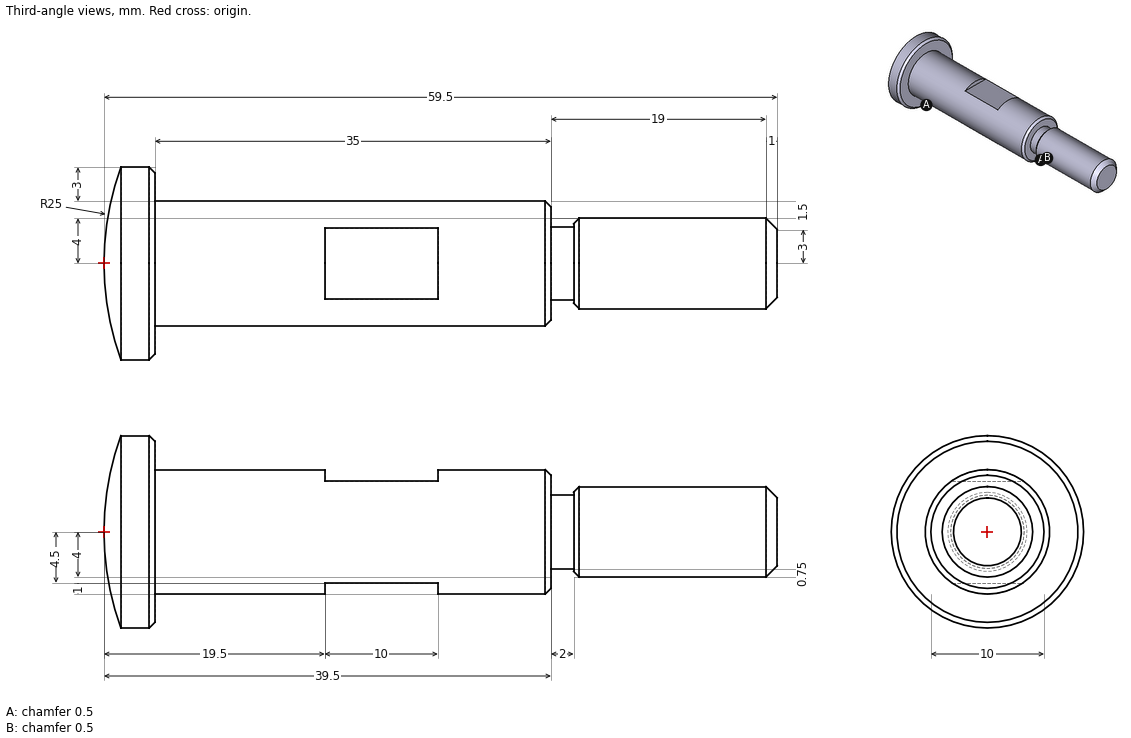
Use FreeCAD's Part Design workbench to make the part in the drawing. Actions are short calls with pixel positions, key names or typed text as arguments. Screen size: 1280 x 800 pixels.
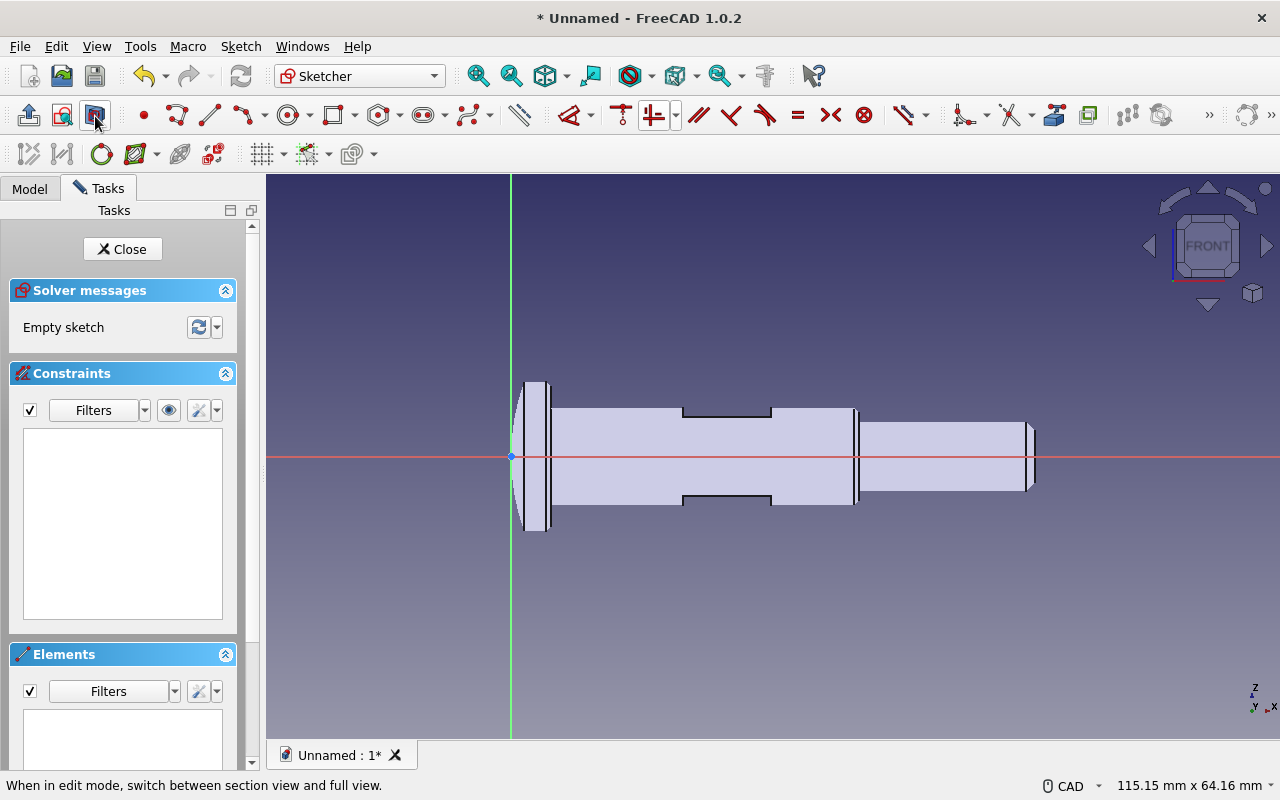
scroll(876, 490, up, 15)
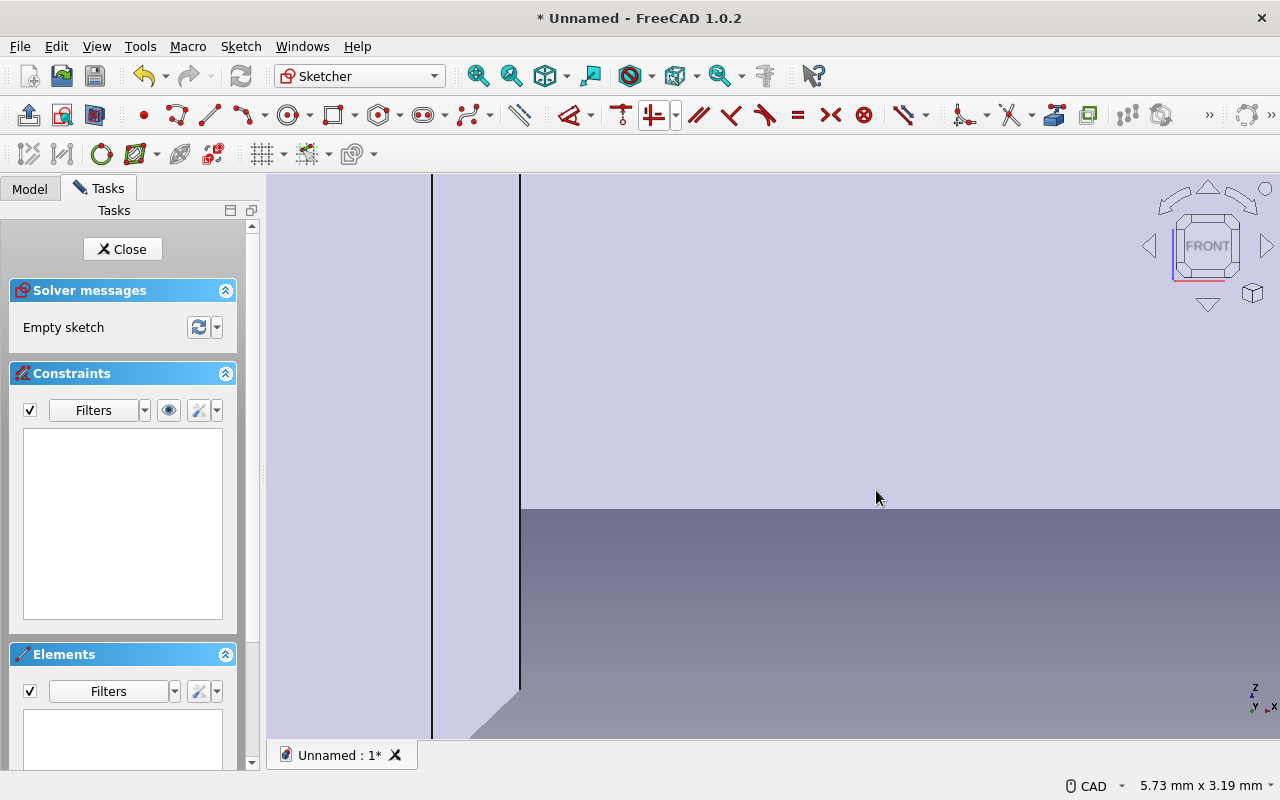
scroll(682, 430, up, 2)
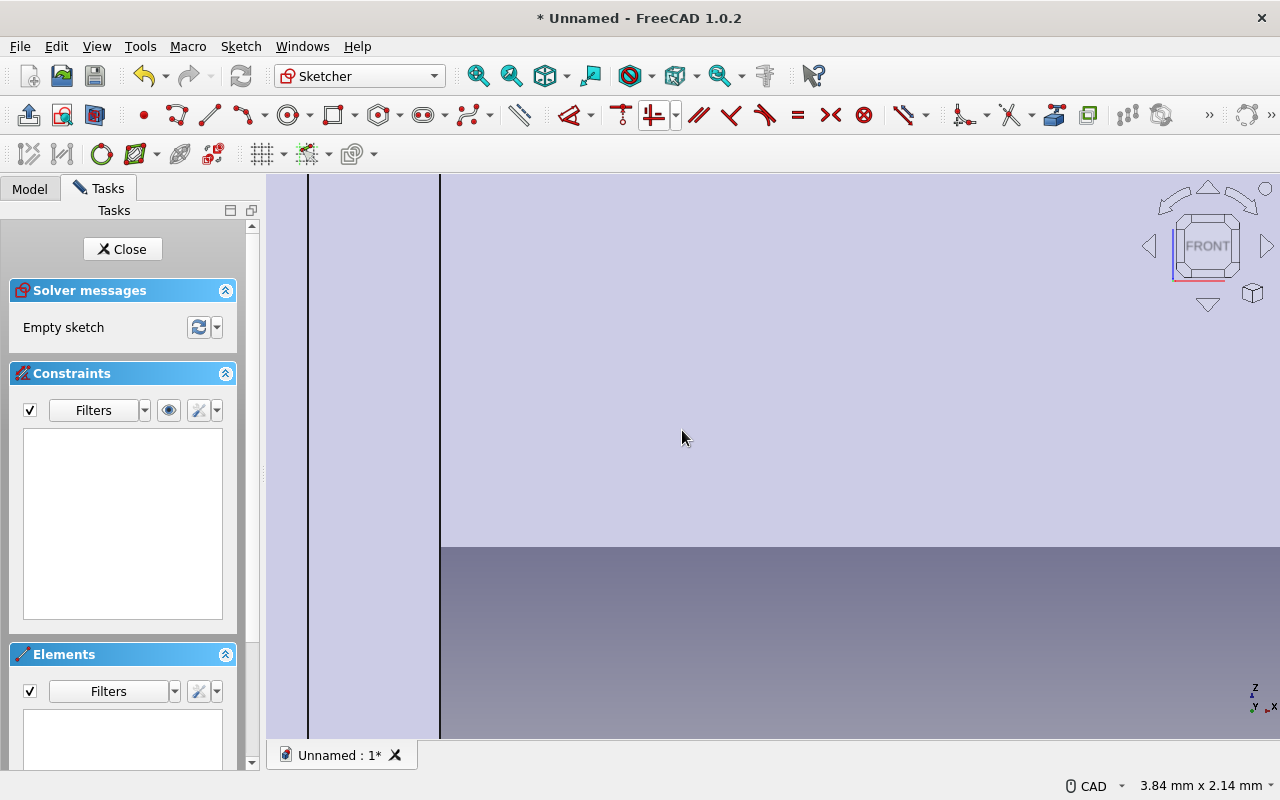
click(332, 116)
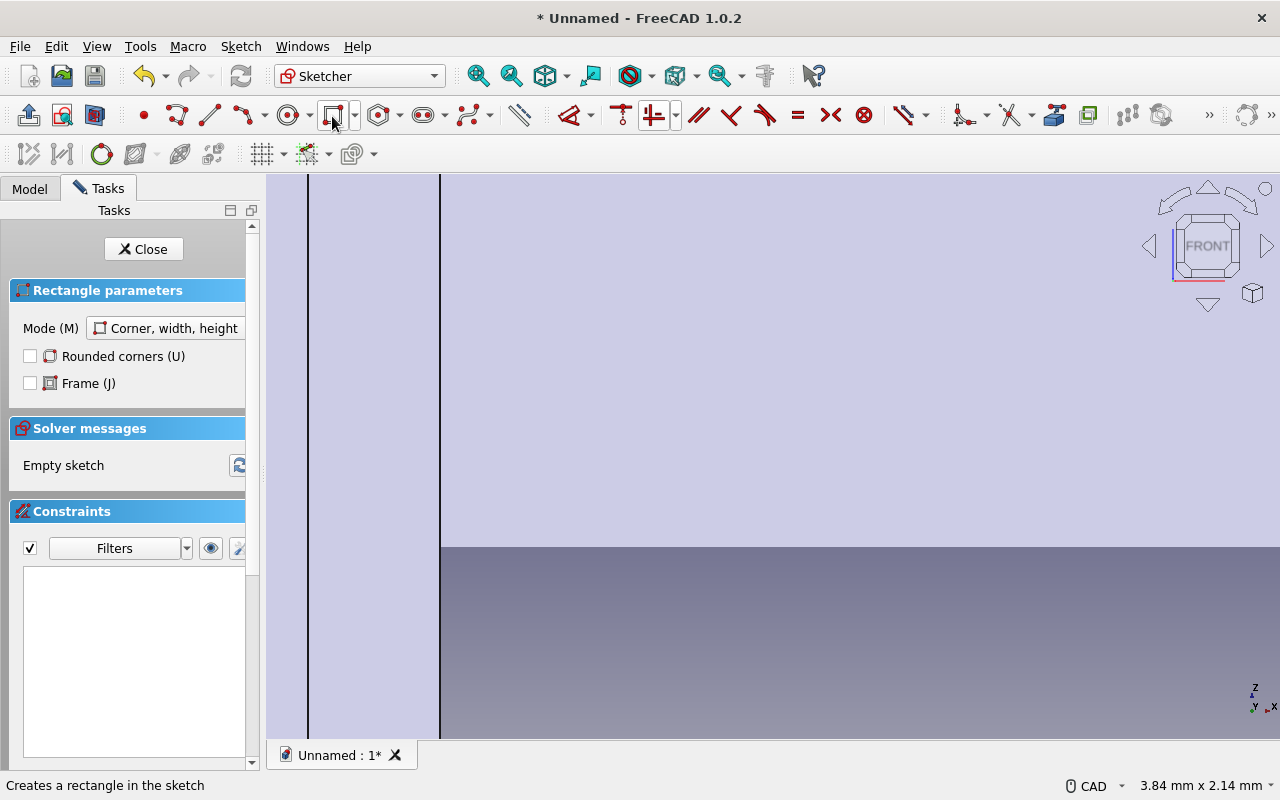
click(440, 357)
move(968, 555)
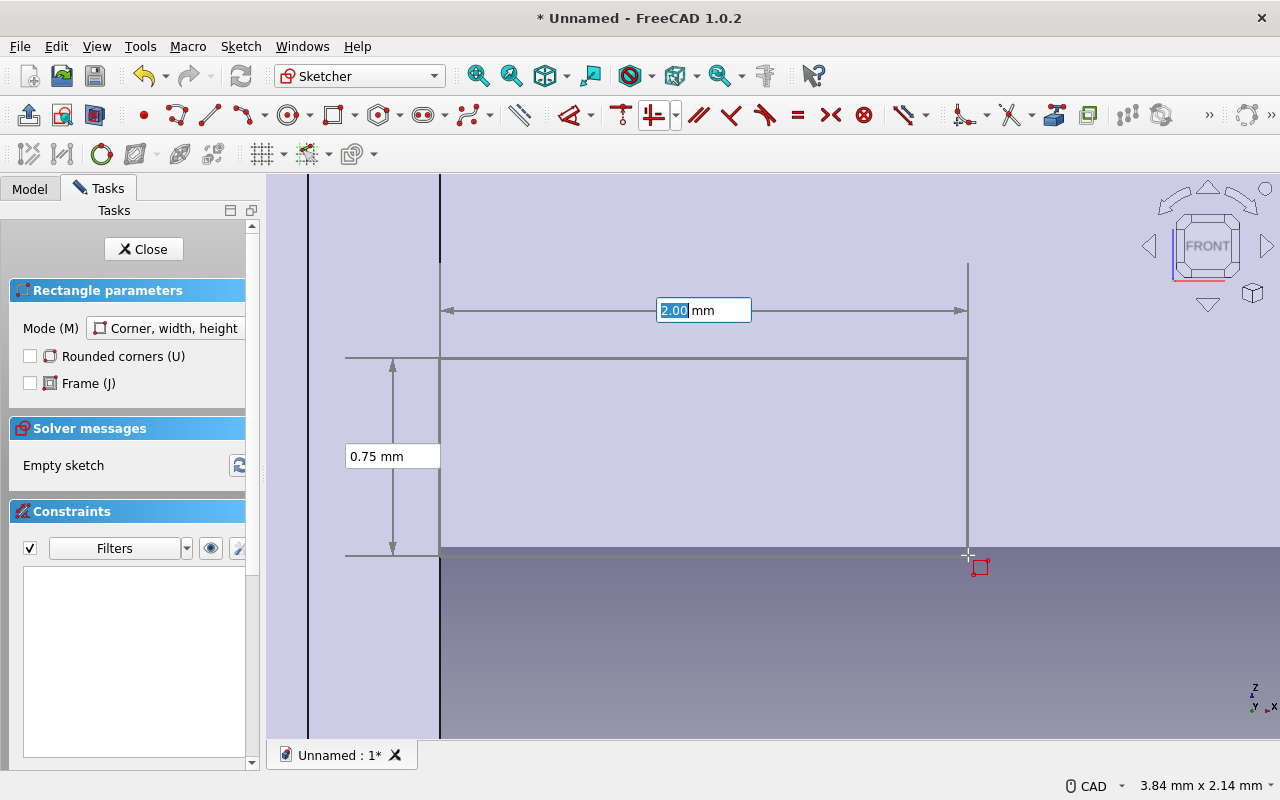
text(2)
key(Tab)
text(0.75)
key(Return)
key(Escape)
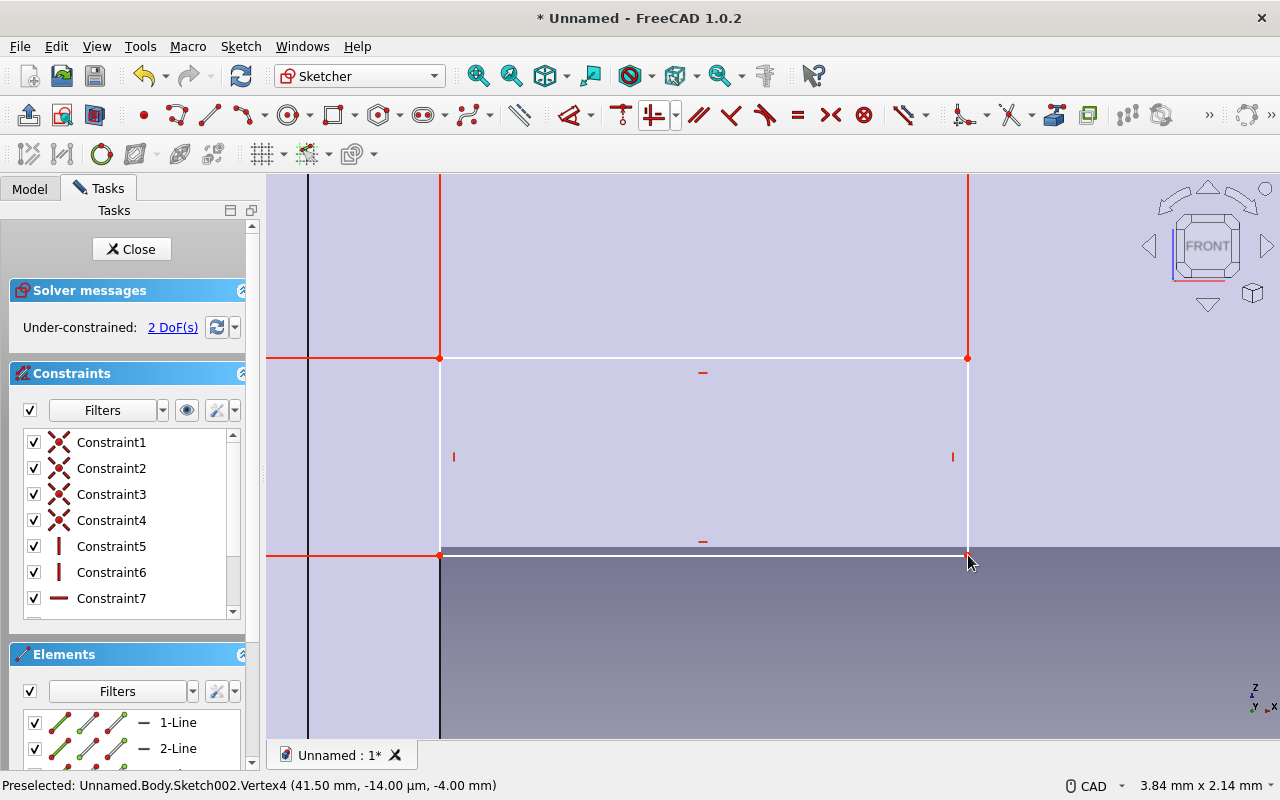
click(568, 116)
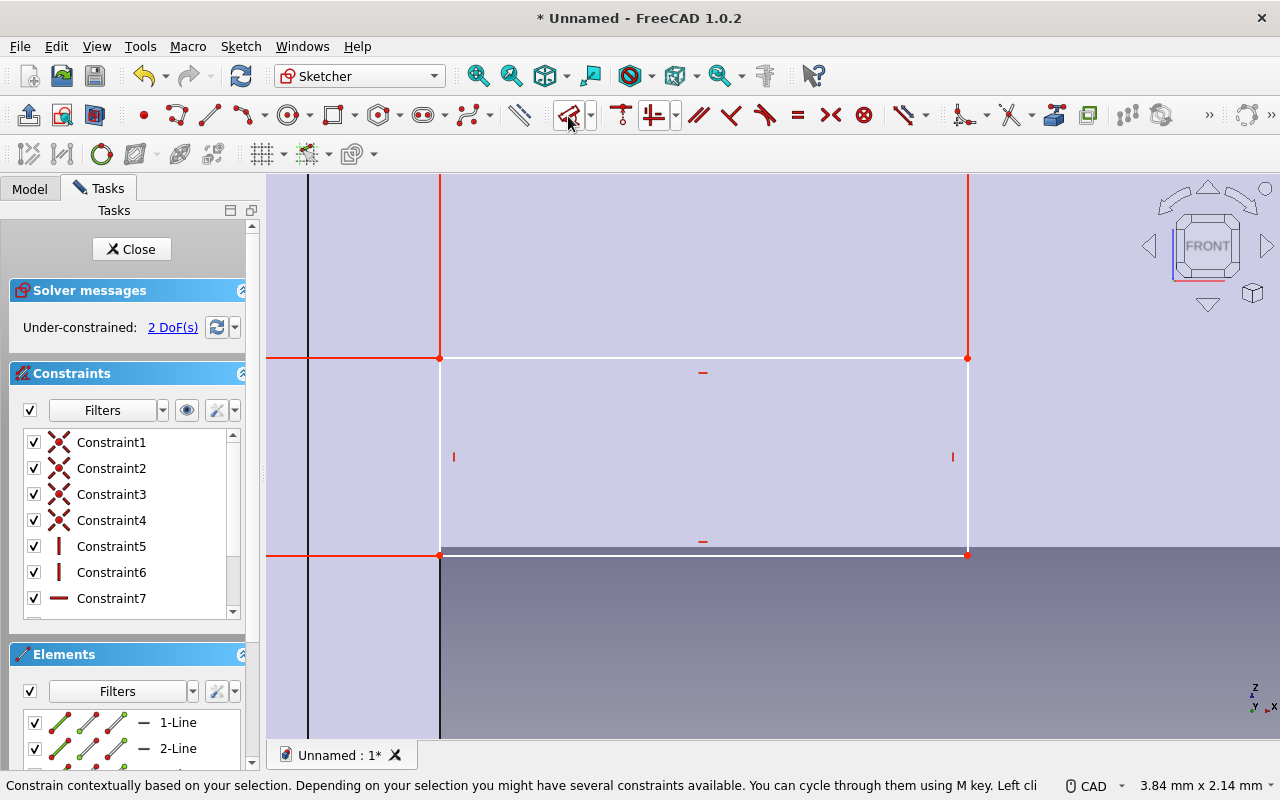
click(440, 556)
click(474, 379)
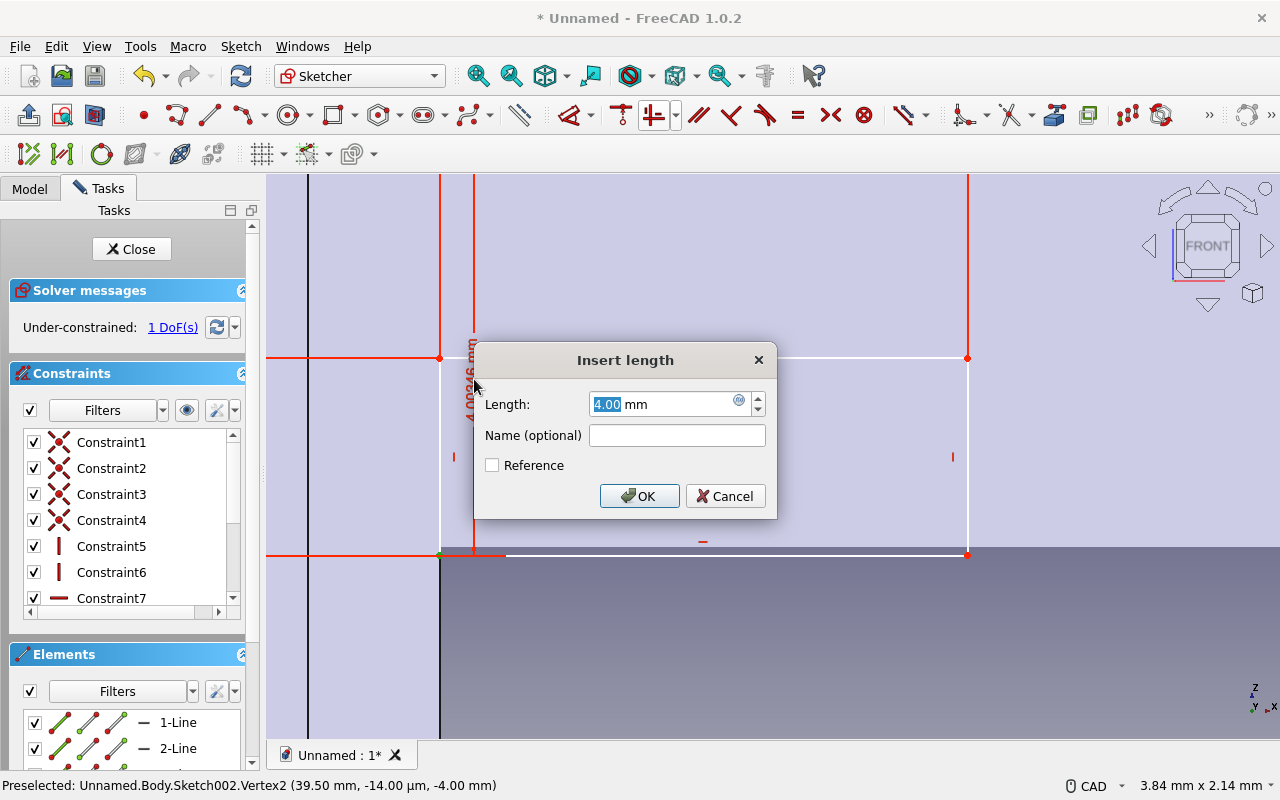
text(4)
key(Return)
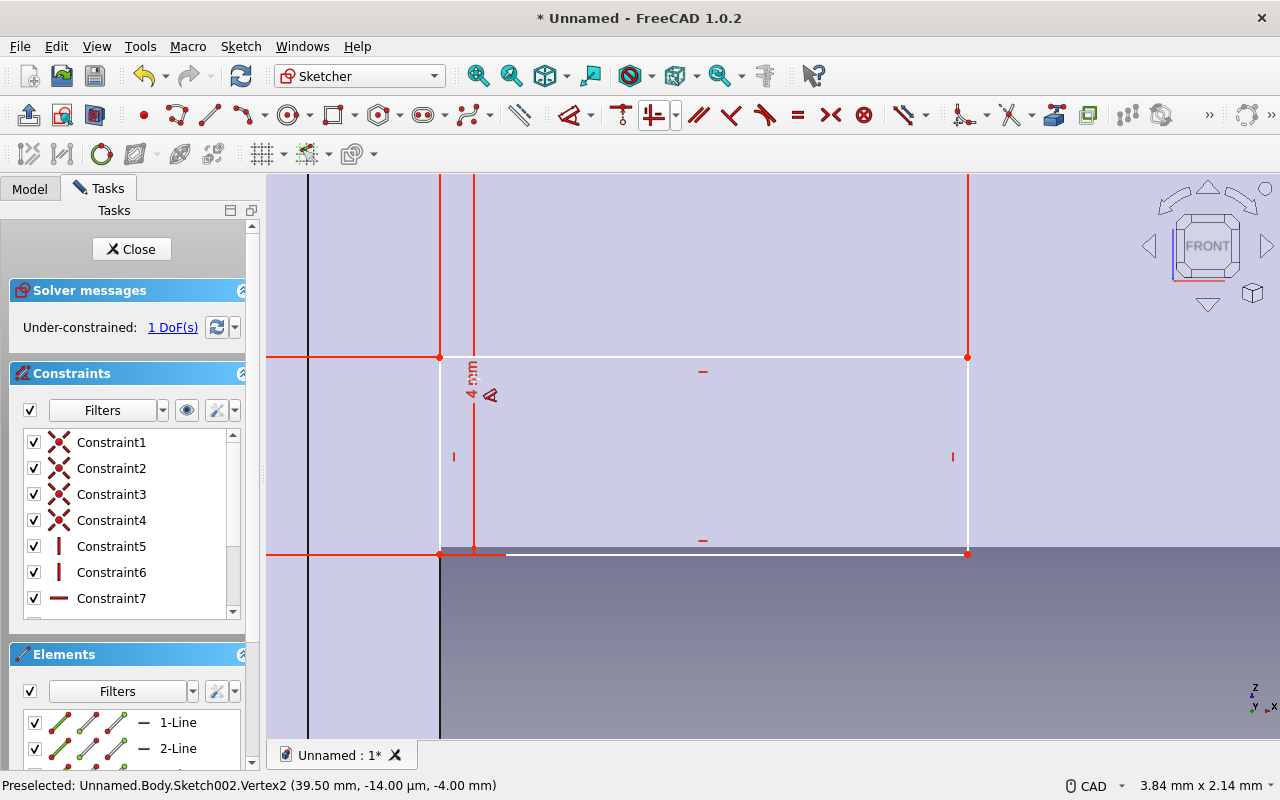
click(440, 357)
click(367, 391)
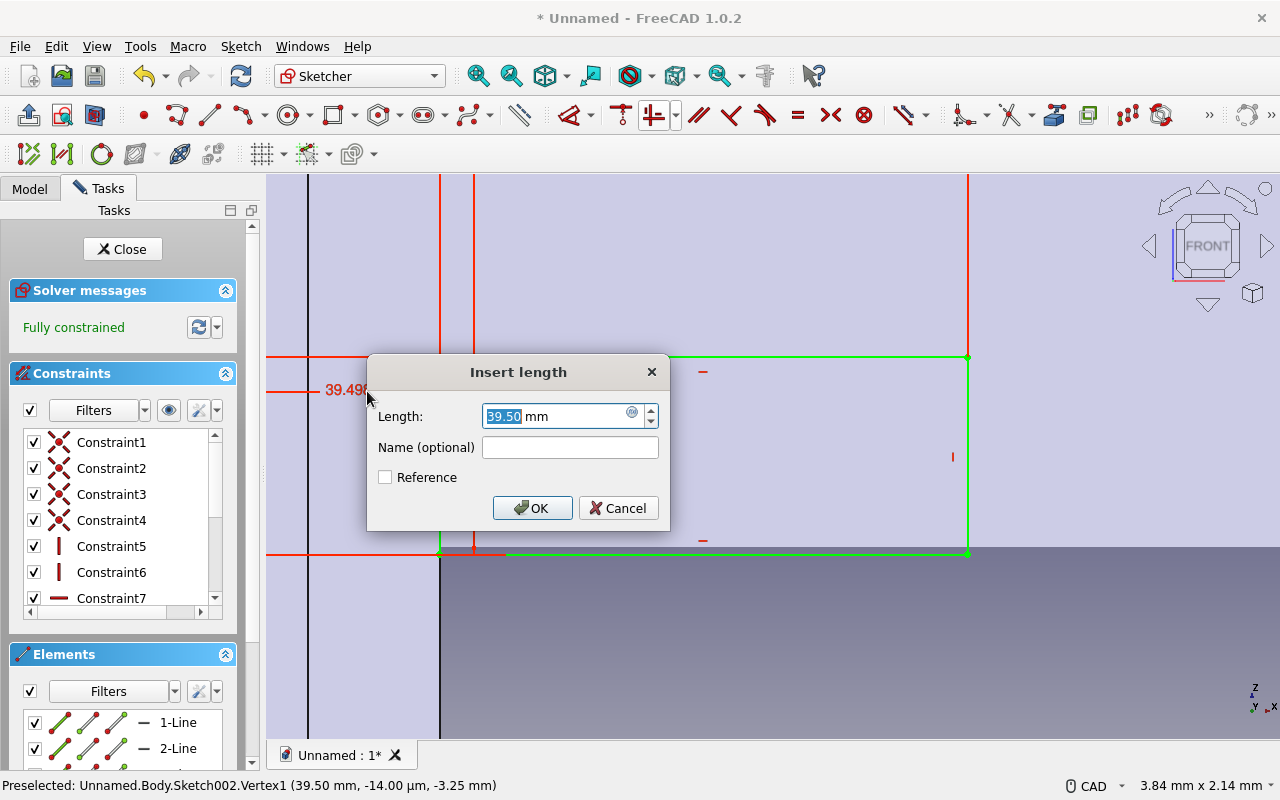
text(39.5)
key(Return)
key(Escape)